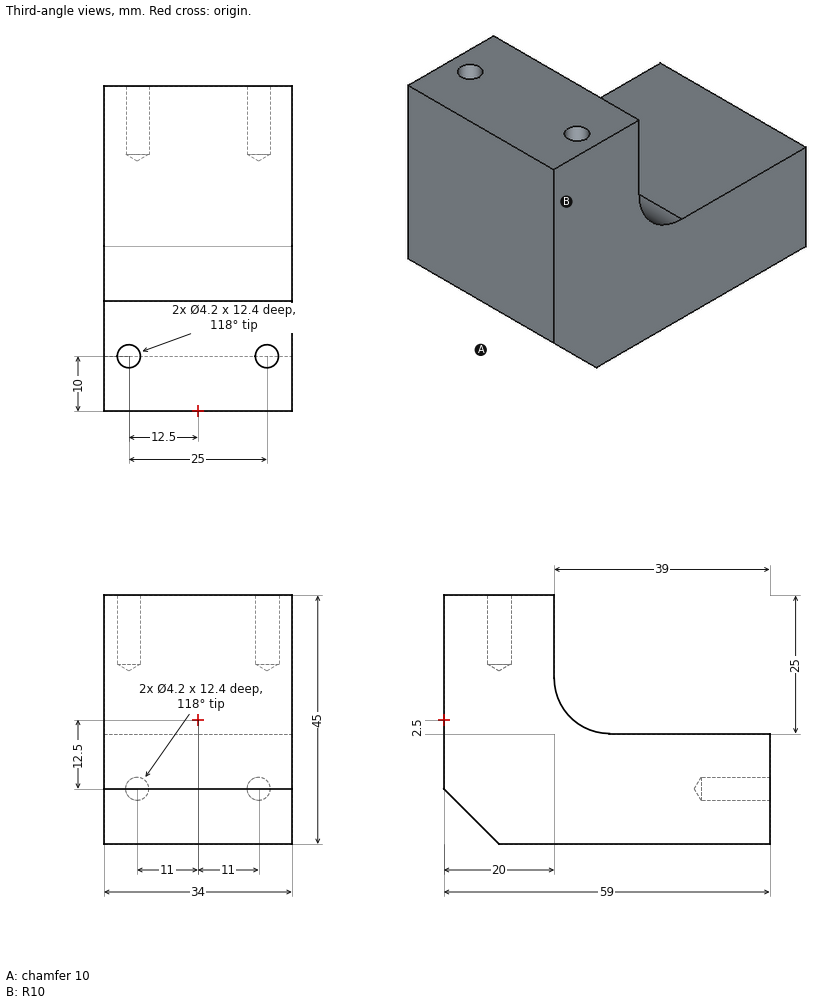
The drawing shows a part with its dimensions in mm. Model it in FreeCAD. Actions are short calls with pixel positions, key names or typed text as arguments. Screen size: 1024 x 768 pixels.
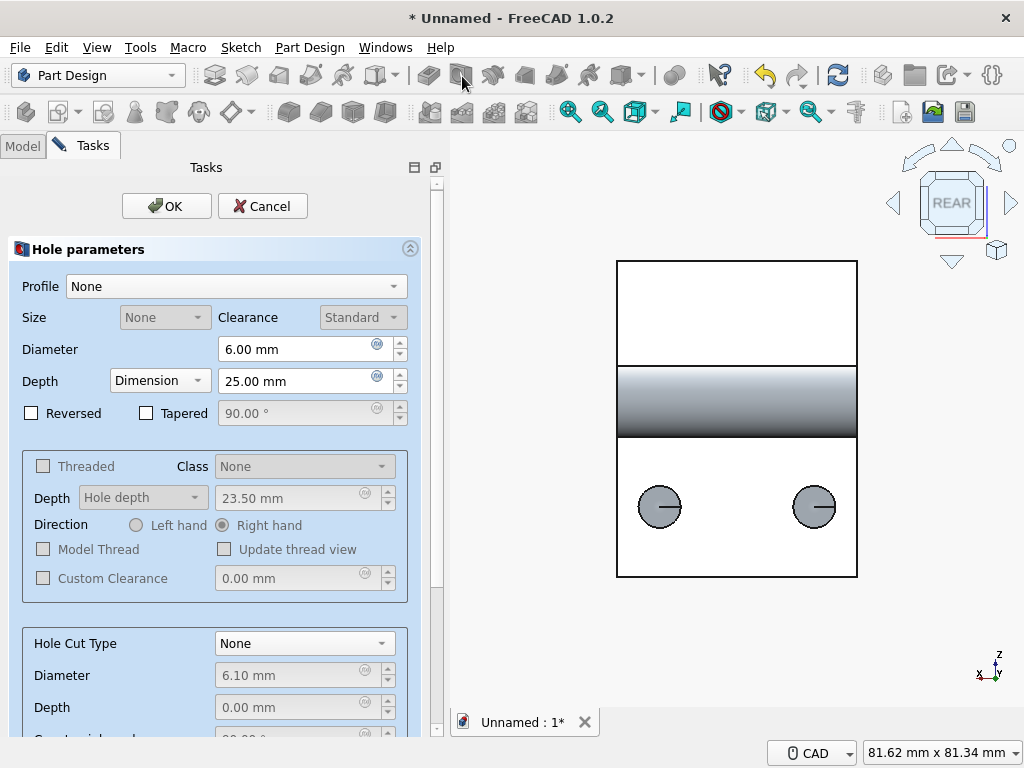
triple_click(305, 349)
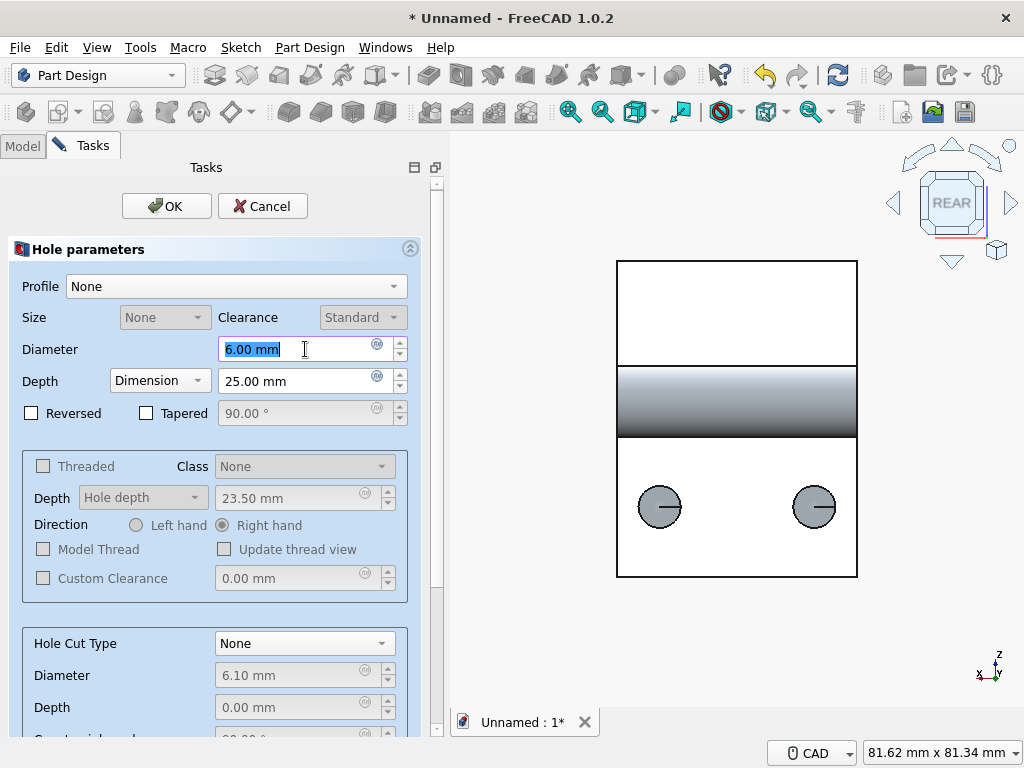
text(4.2)
key(Tab)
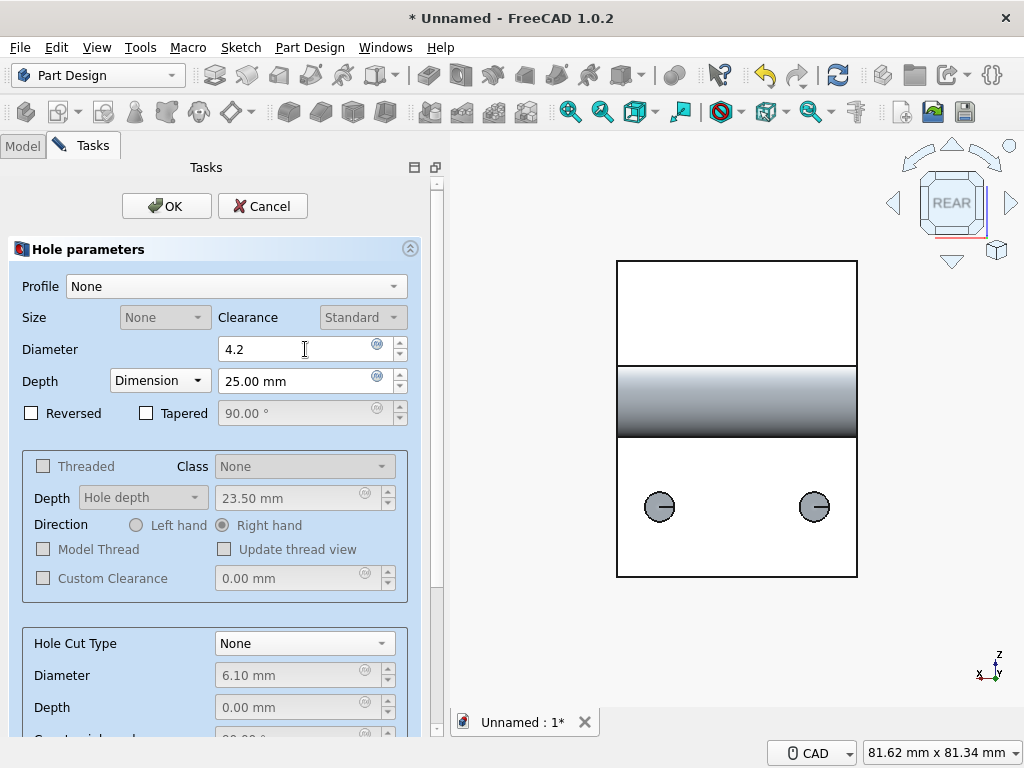
triple_click(305, 381)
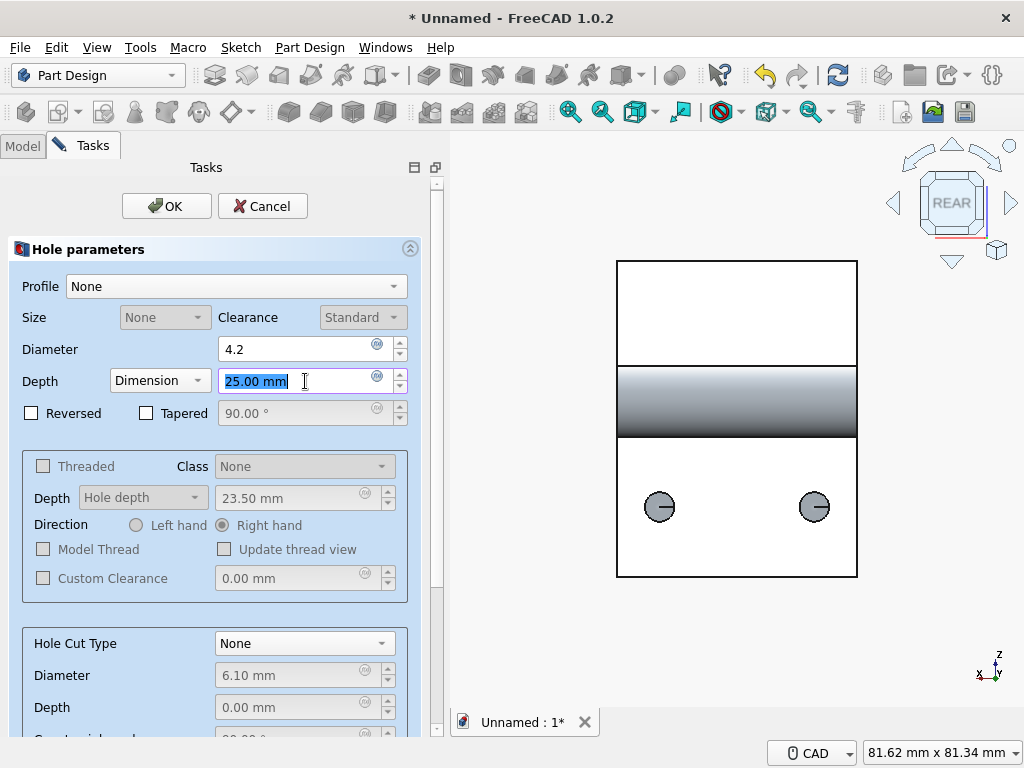
text(12.4)
key(Tab)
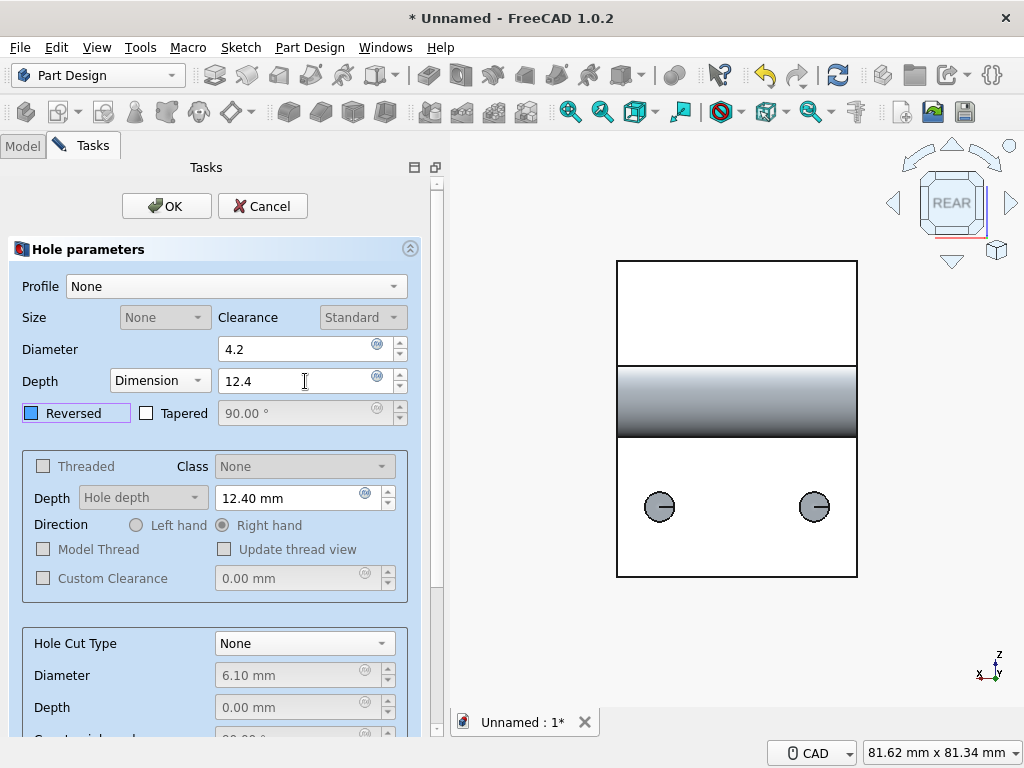
click(167, 206)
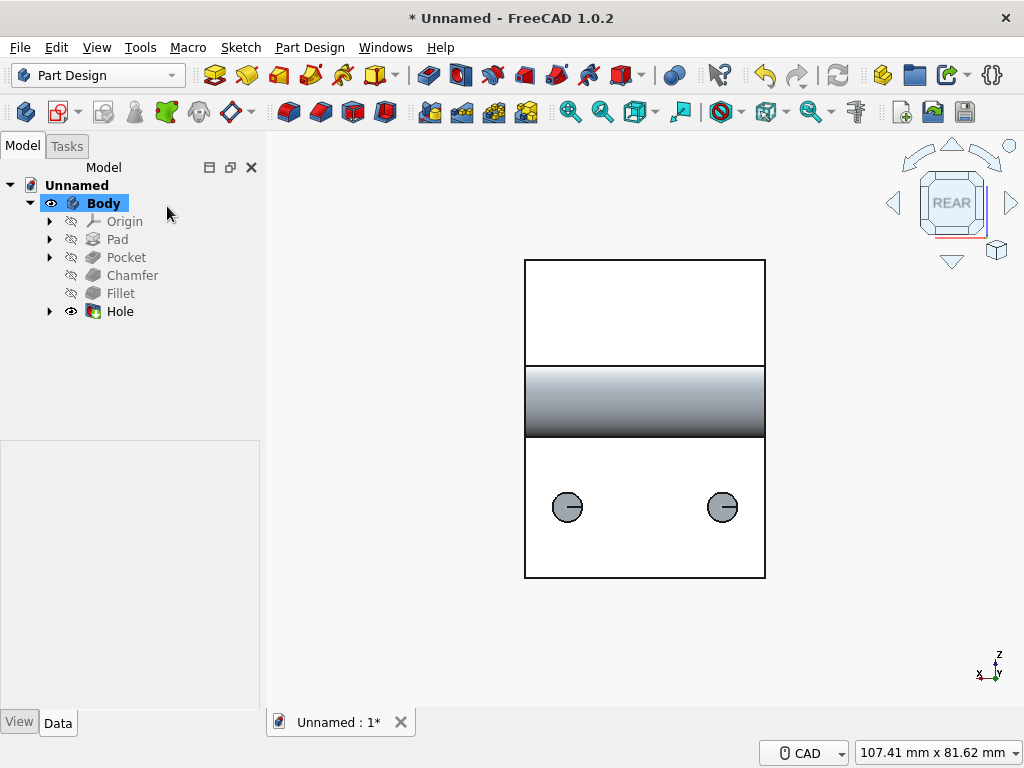
key(0)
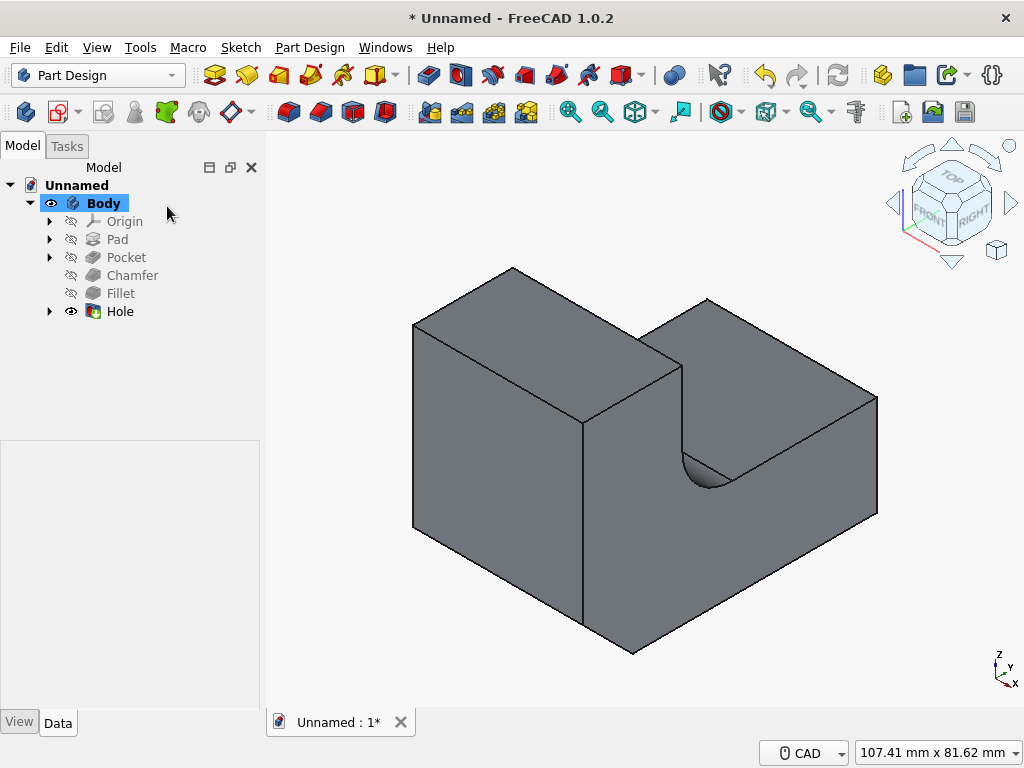
click(572, 359)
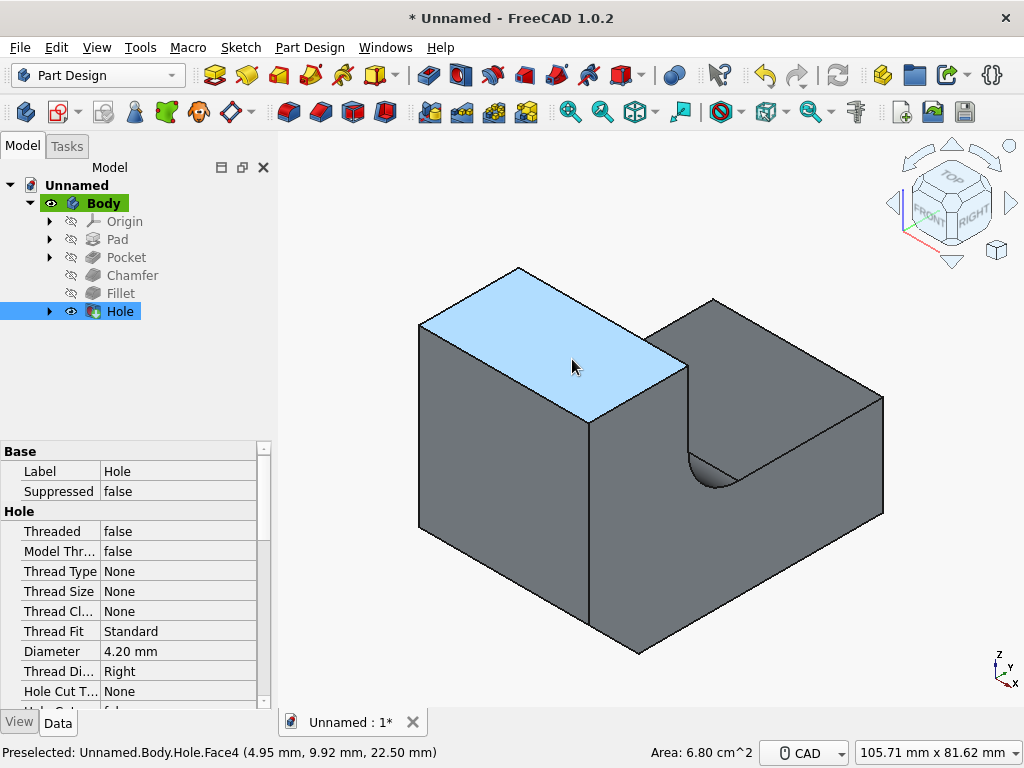
click(58, 112)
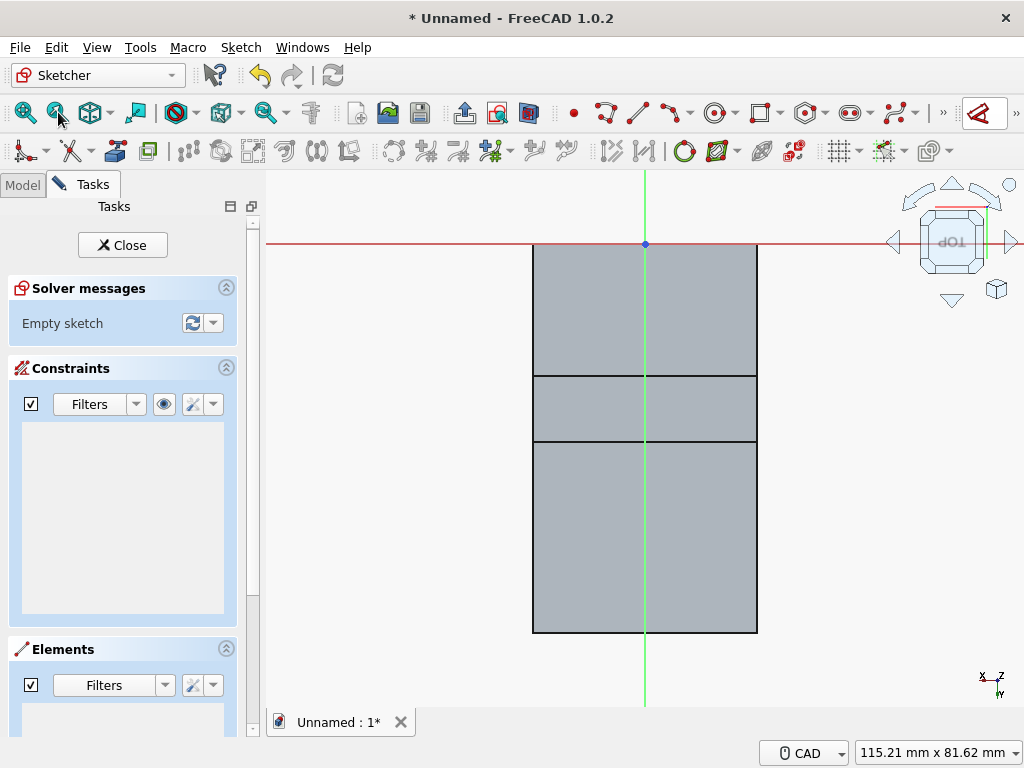
scroll(701, 198, up, 4)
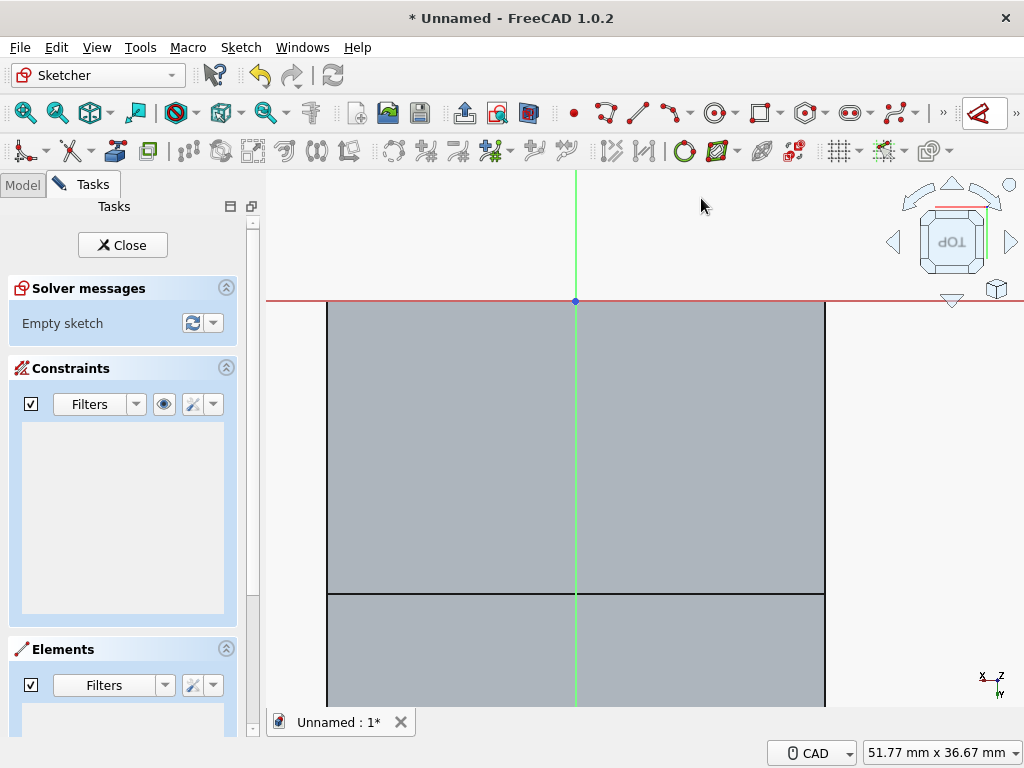
click(716, 114)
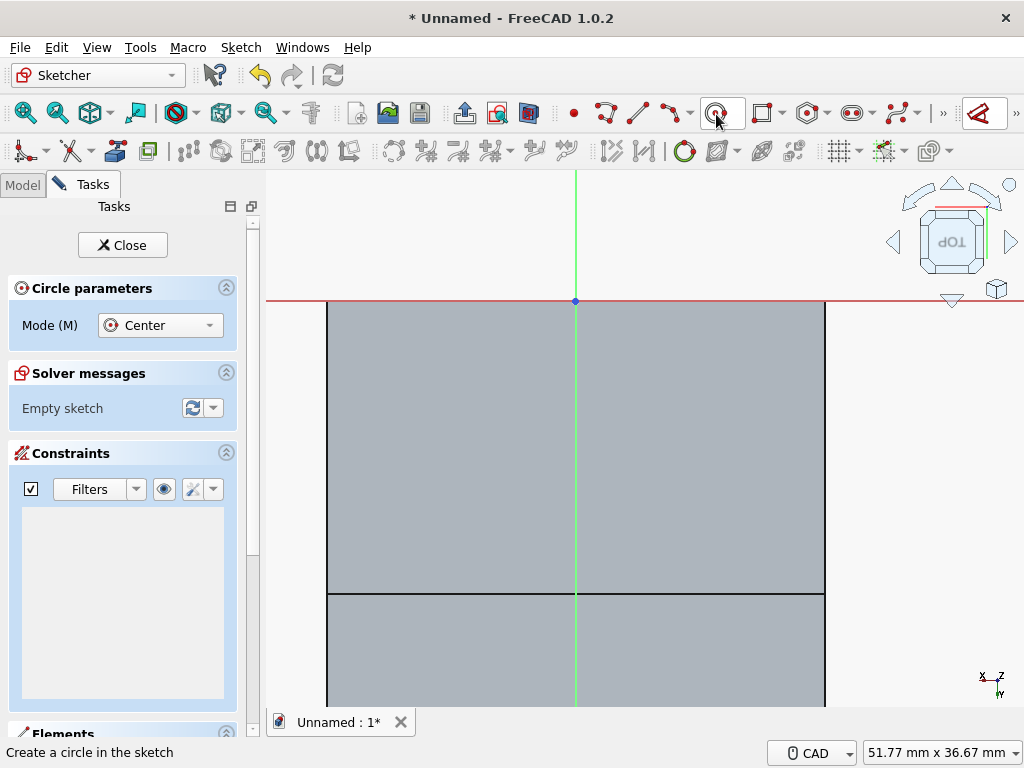
click(759, 448)
move(780, 426)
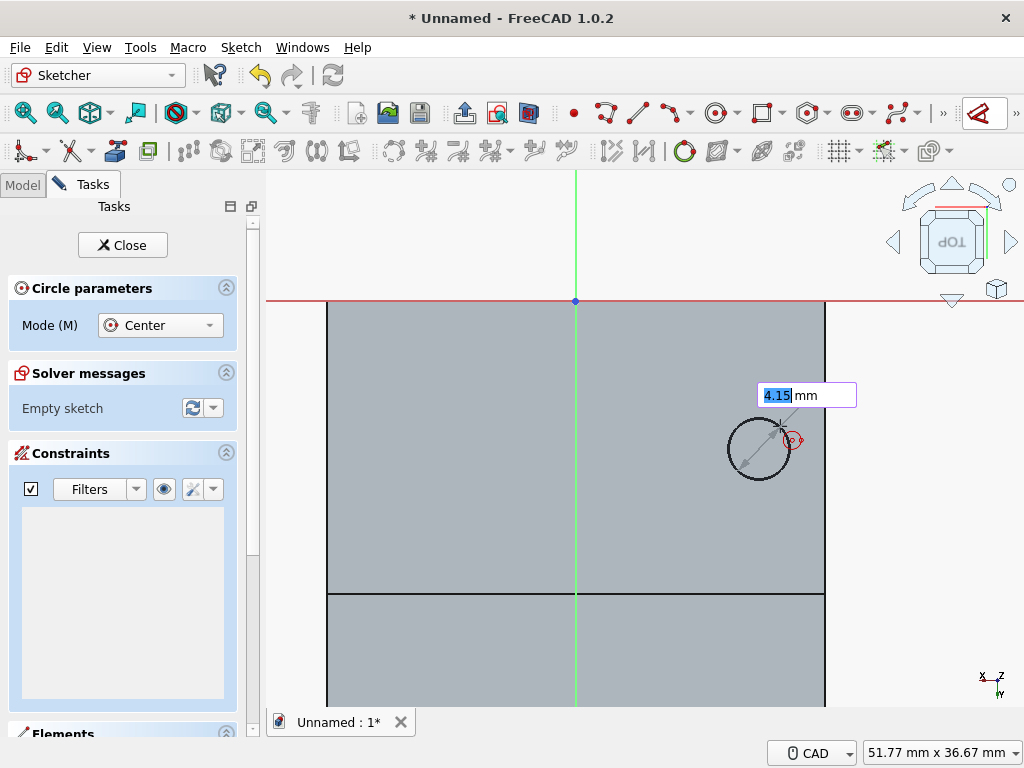
text(4.2)
key(Return)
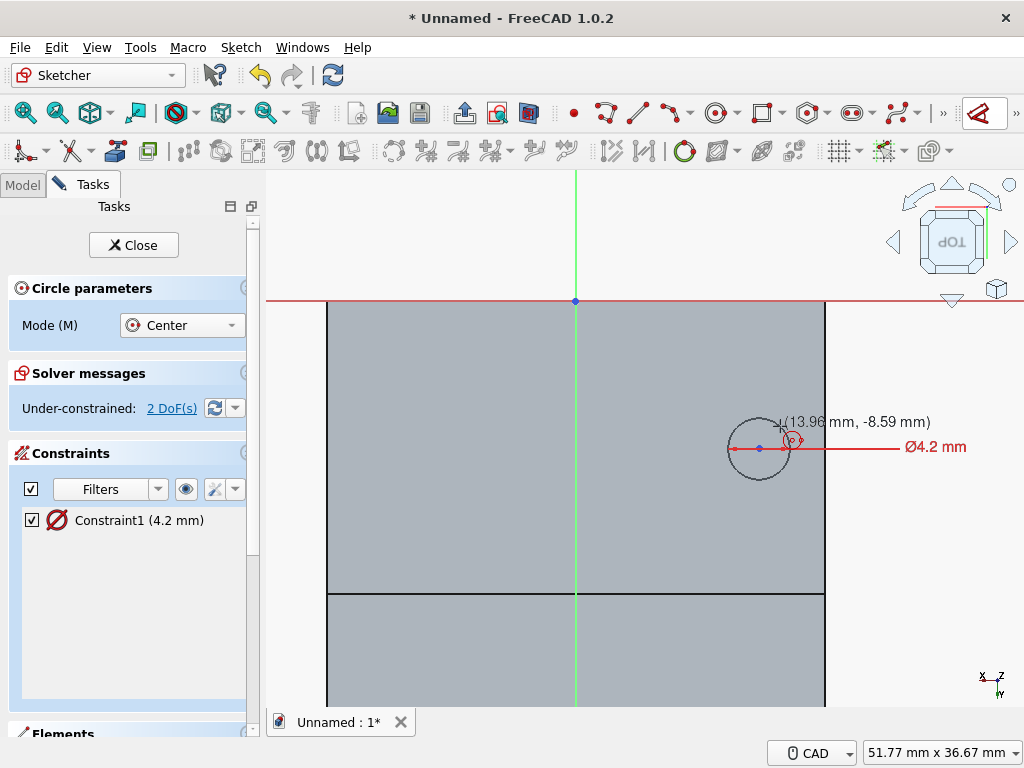
click(393, 448)
move(414, 426)